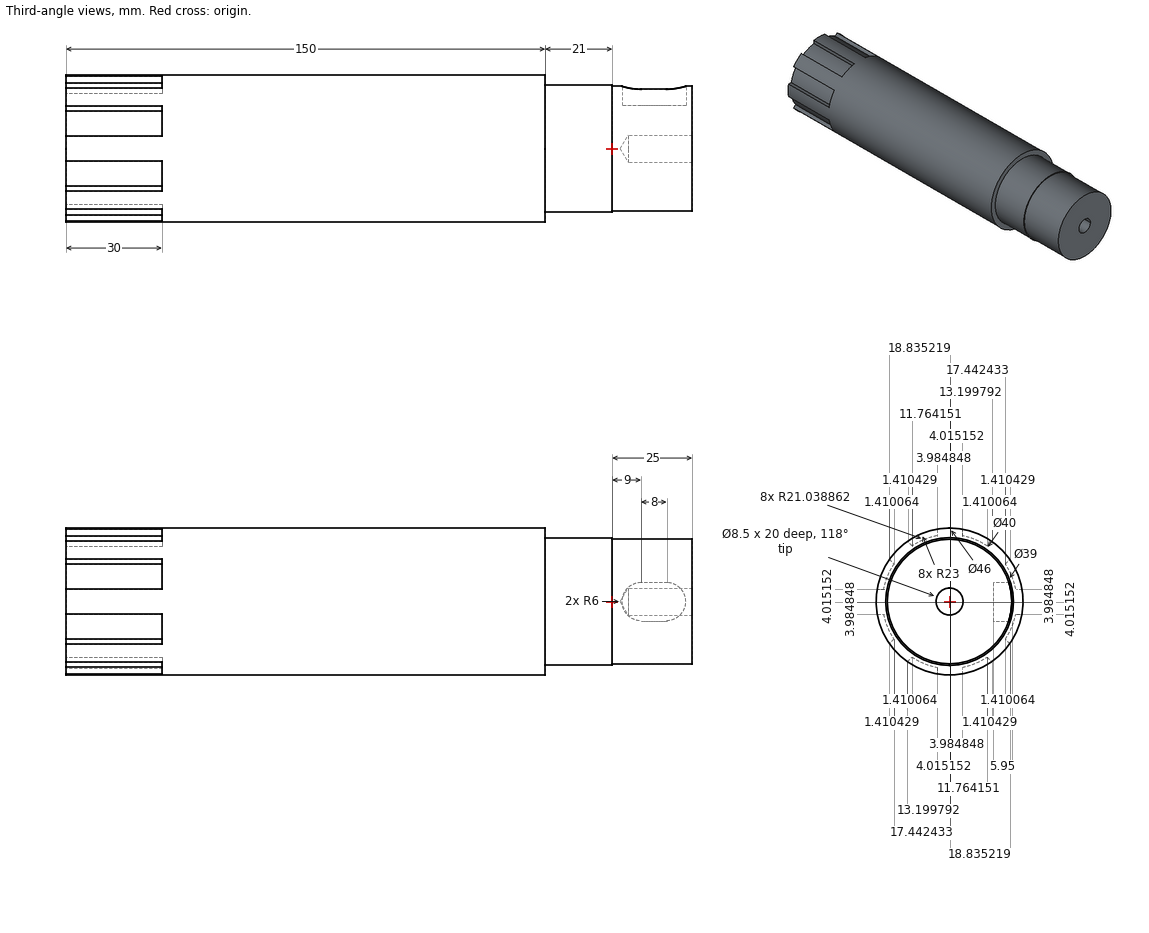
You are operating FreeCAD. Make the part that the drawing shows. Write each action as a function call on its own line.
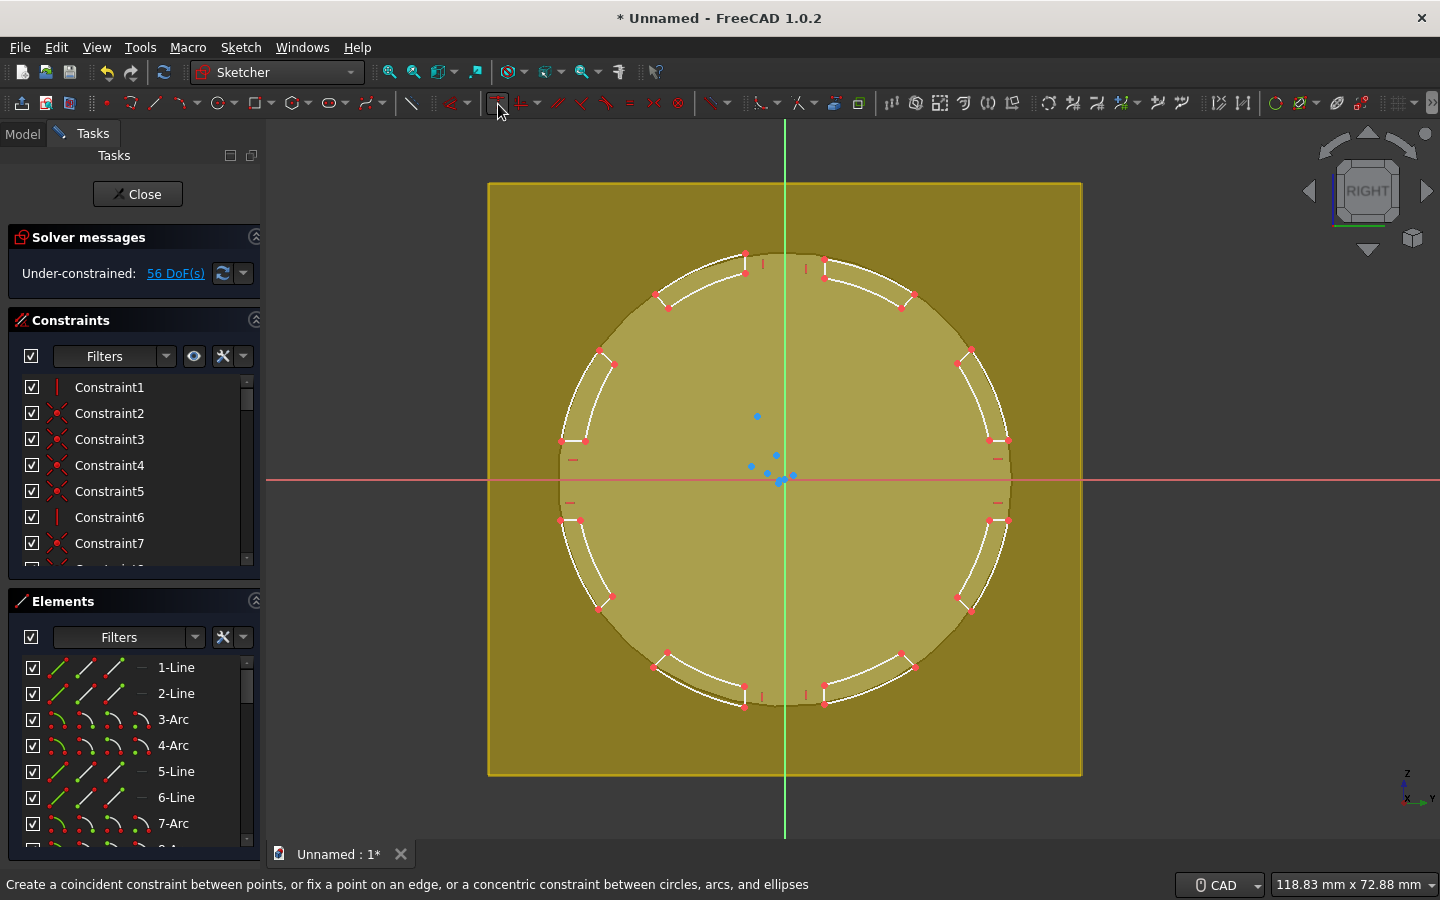
click(721, 280)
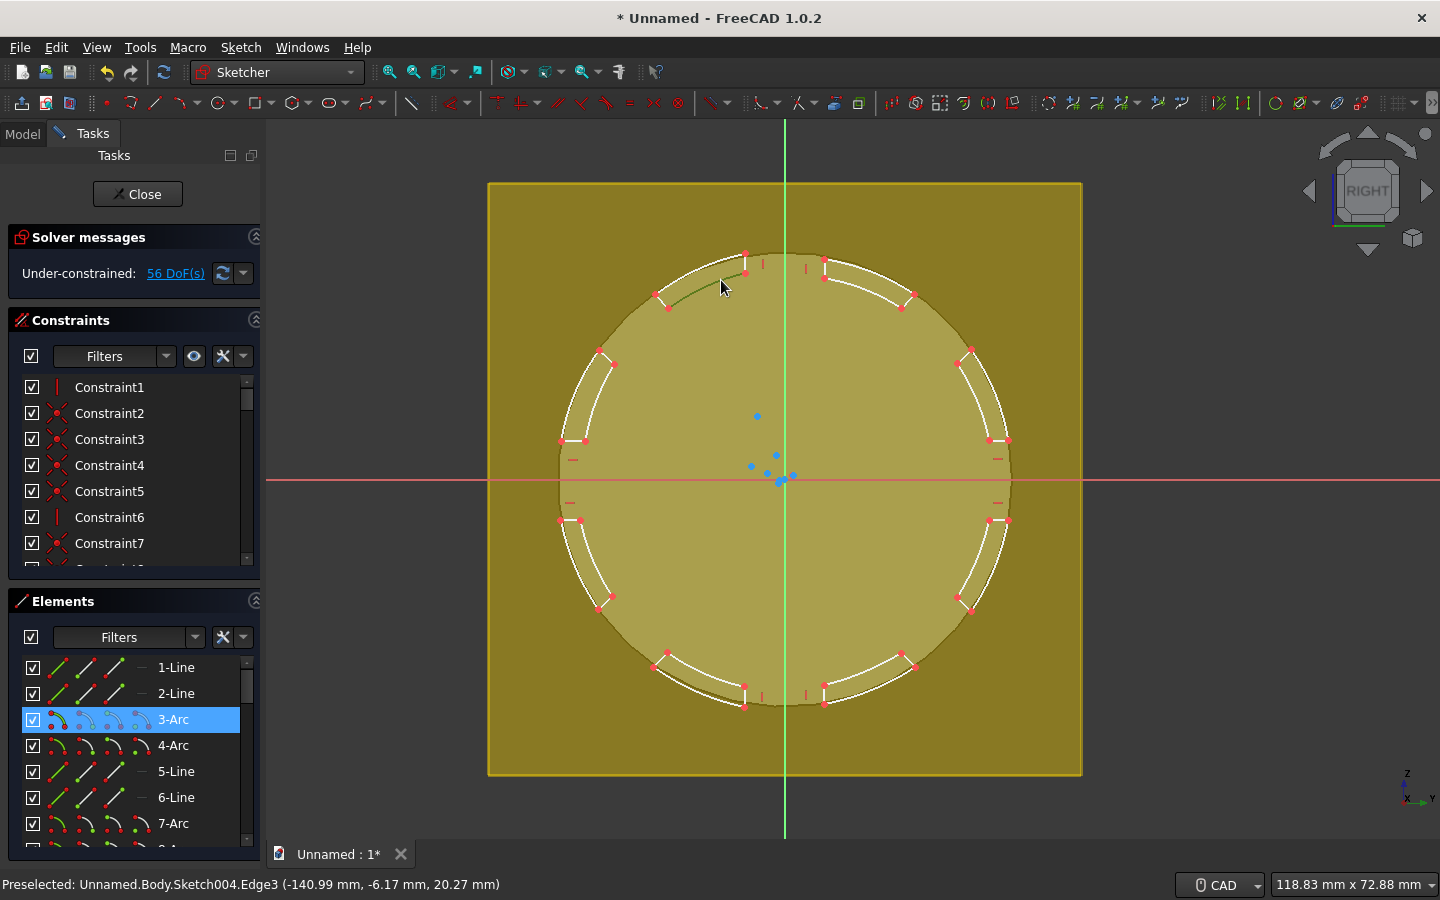
click(583, 376)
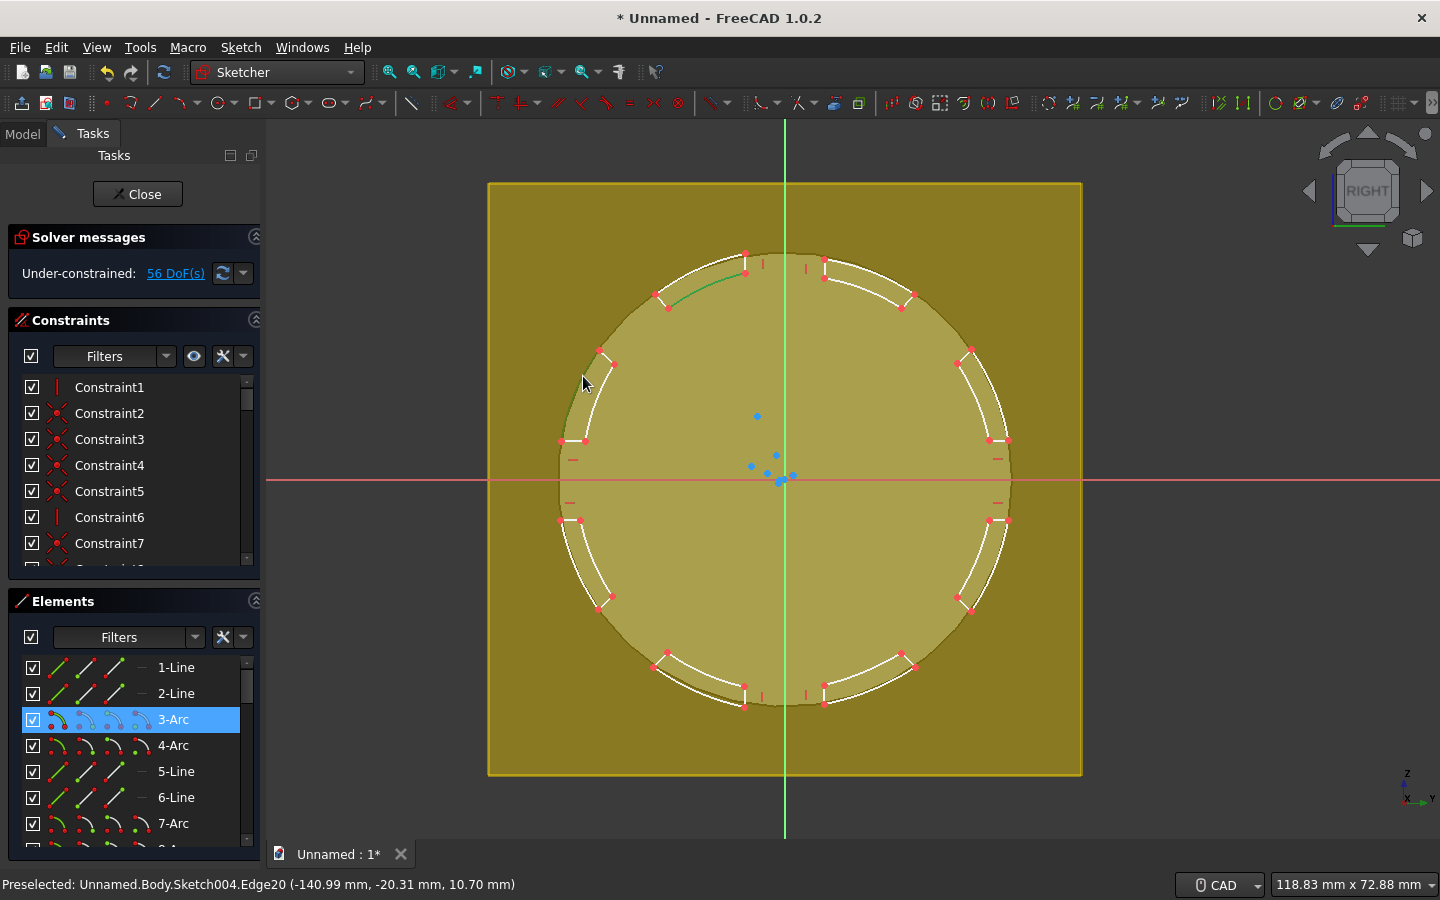
click(498, 104)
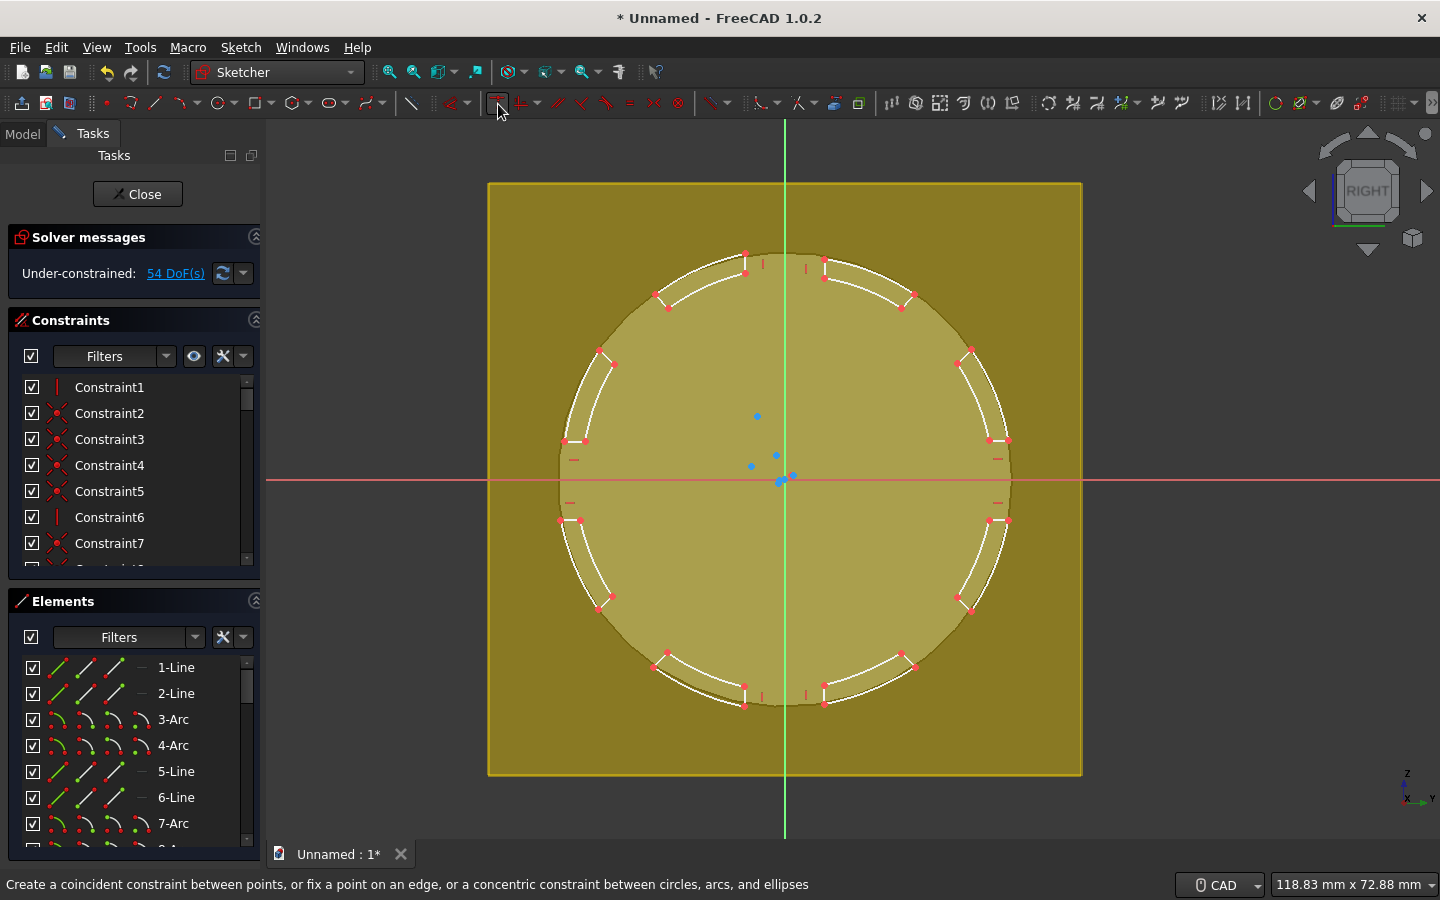
click(721, 281)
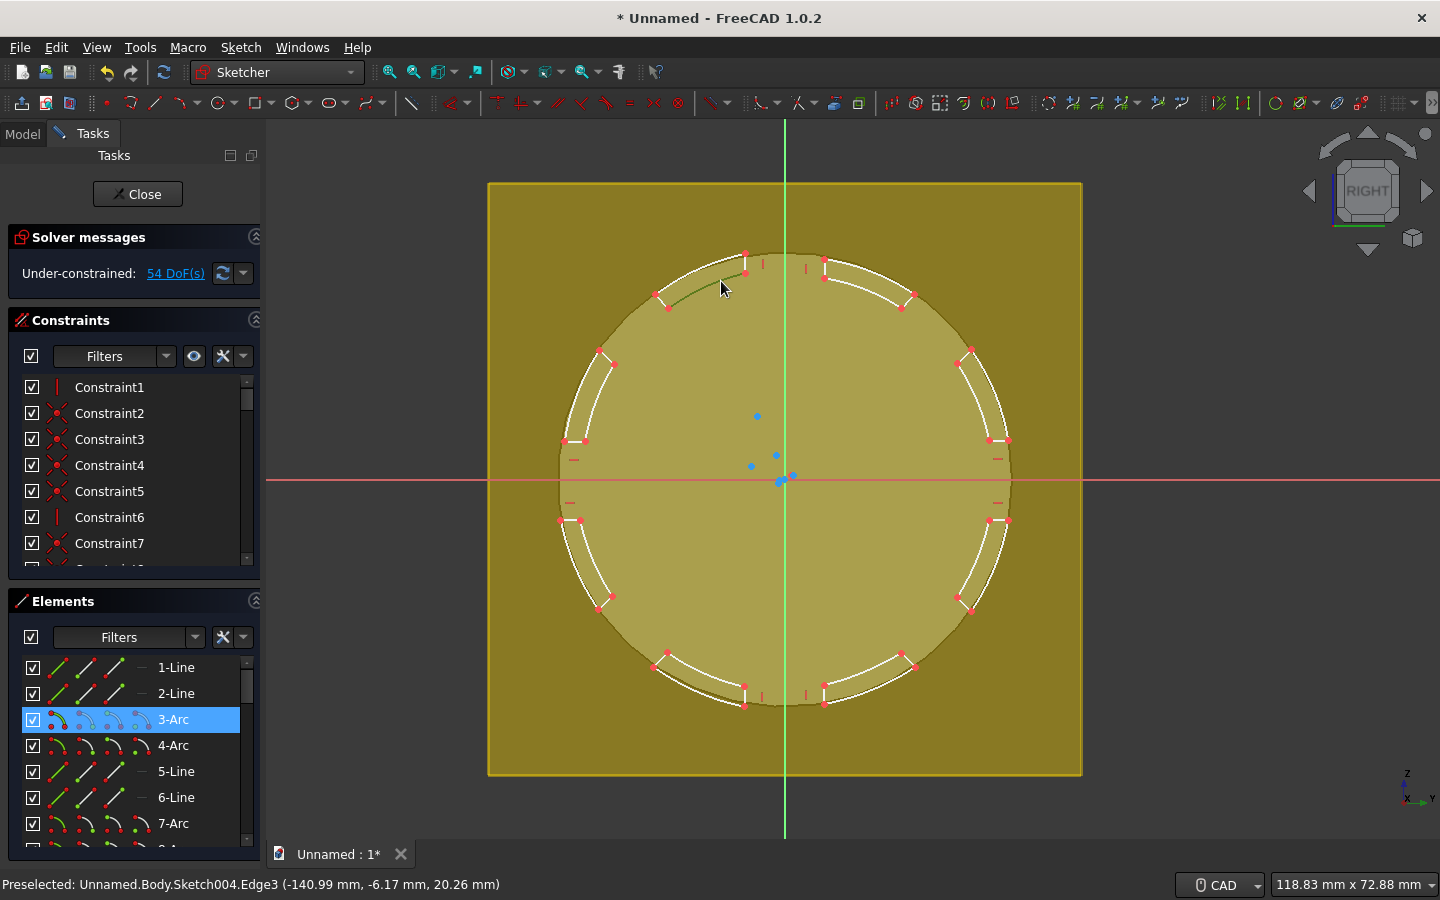
click(983, 417)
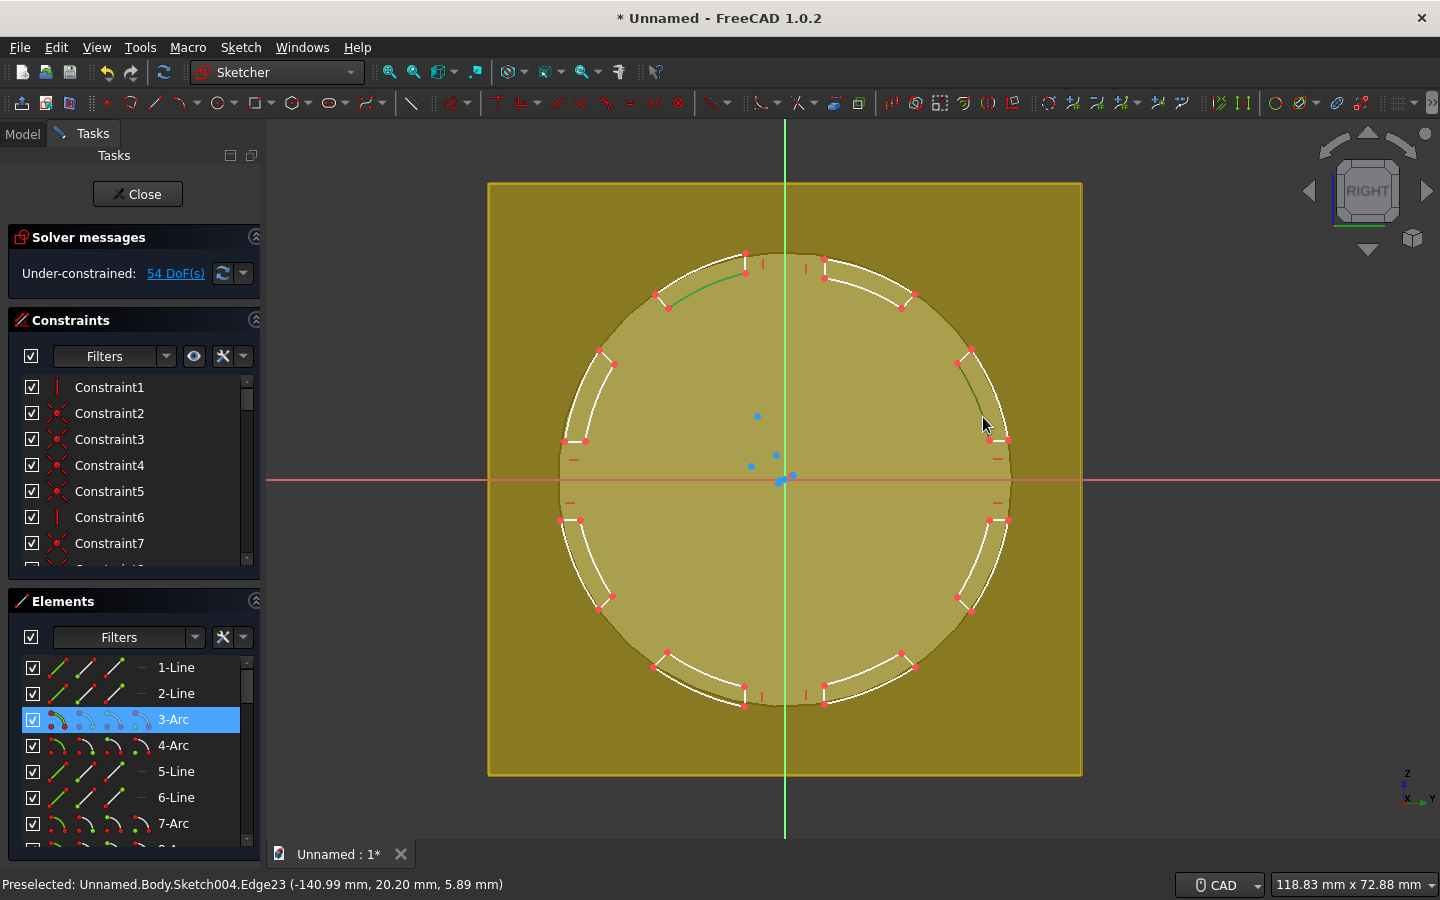
click(498, 104)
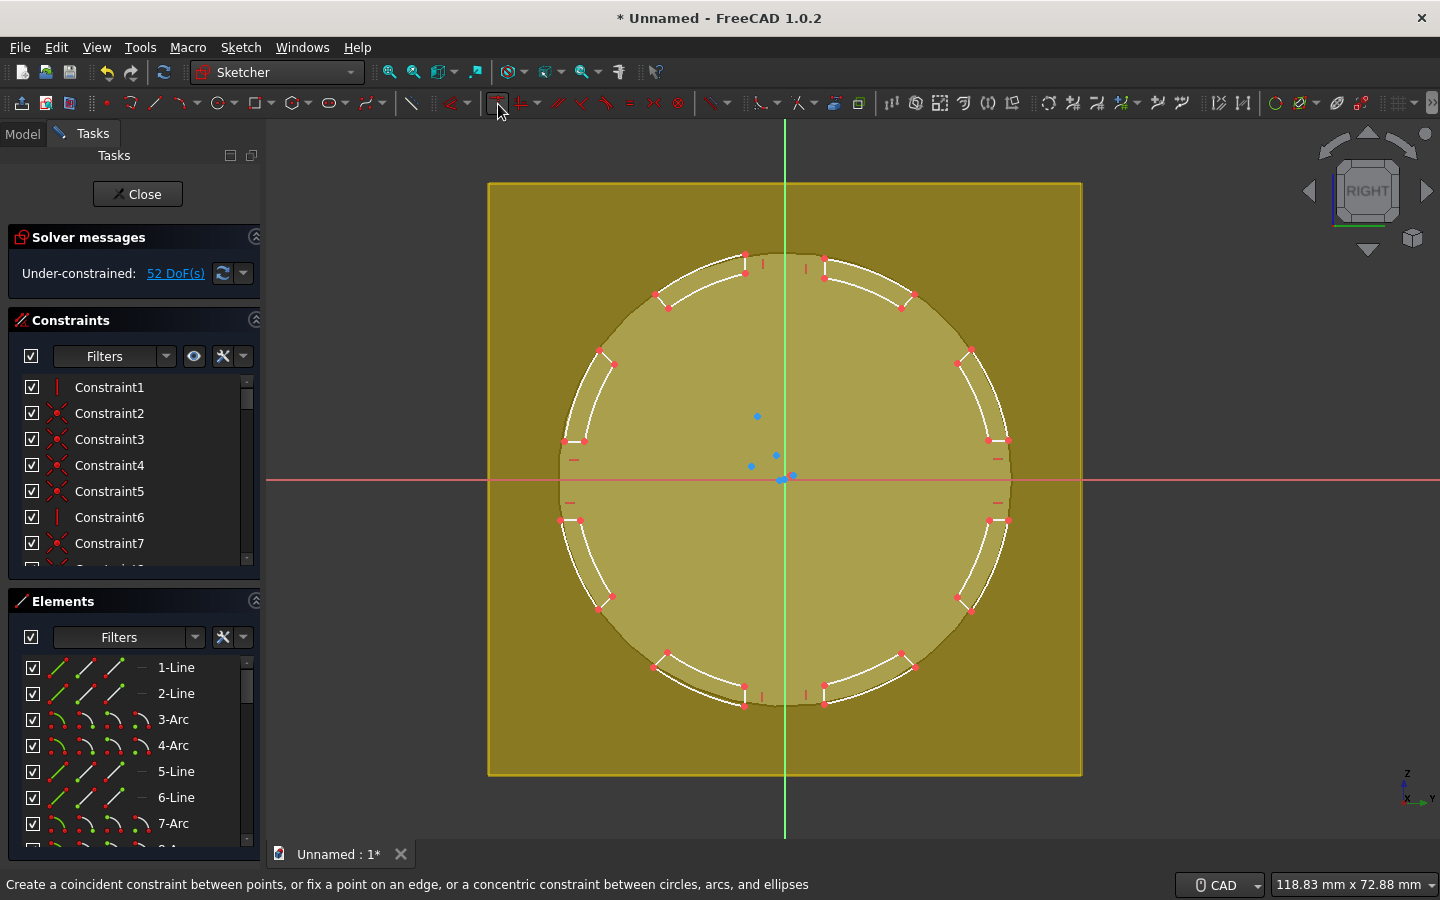
click(721, 281)